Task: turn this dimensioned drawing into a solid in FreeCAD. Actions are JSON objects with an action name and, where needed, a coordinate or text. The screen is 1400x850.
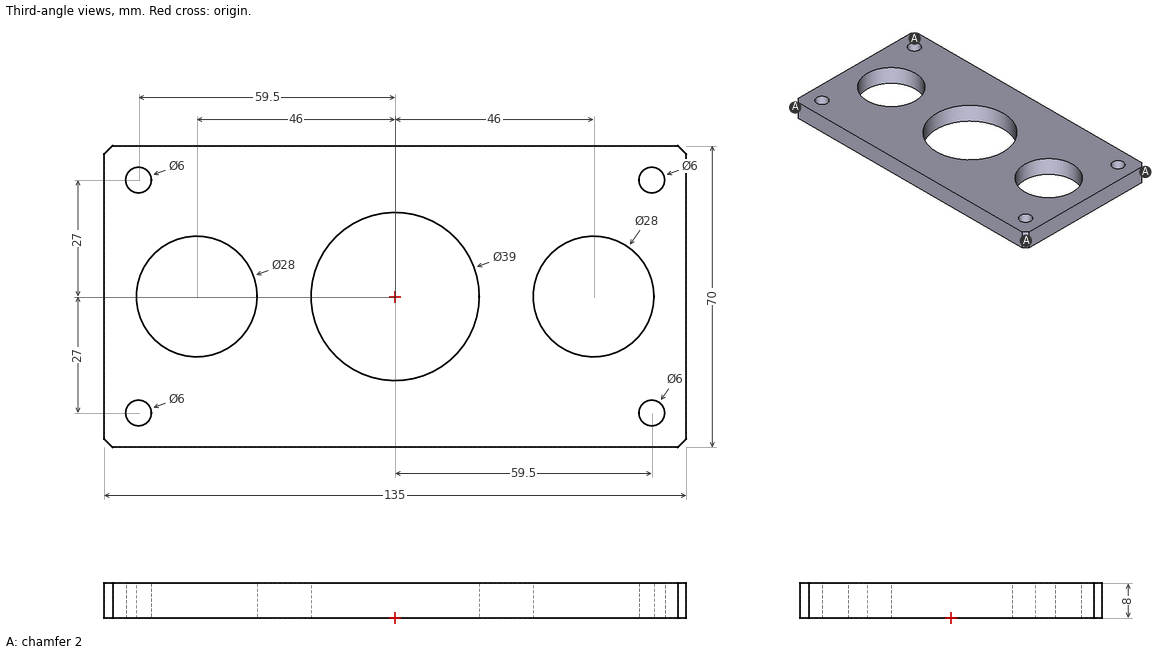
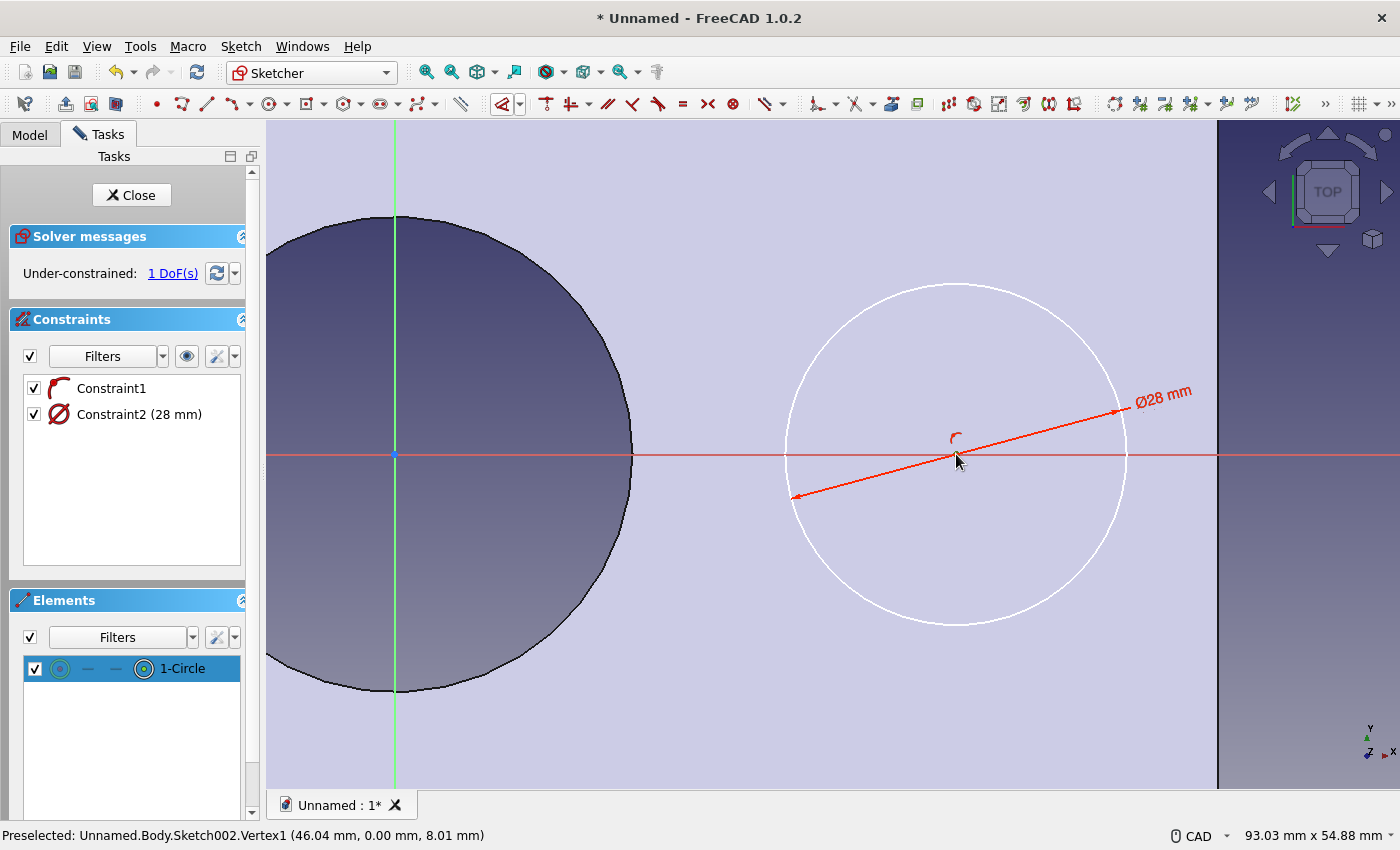
{"action": "key", "text": "l"}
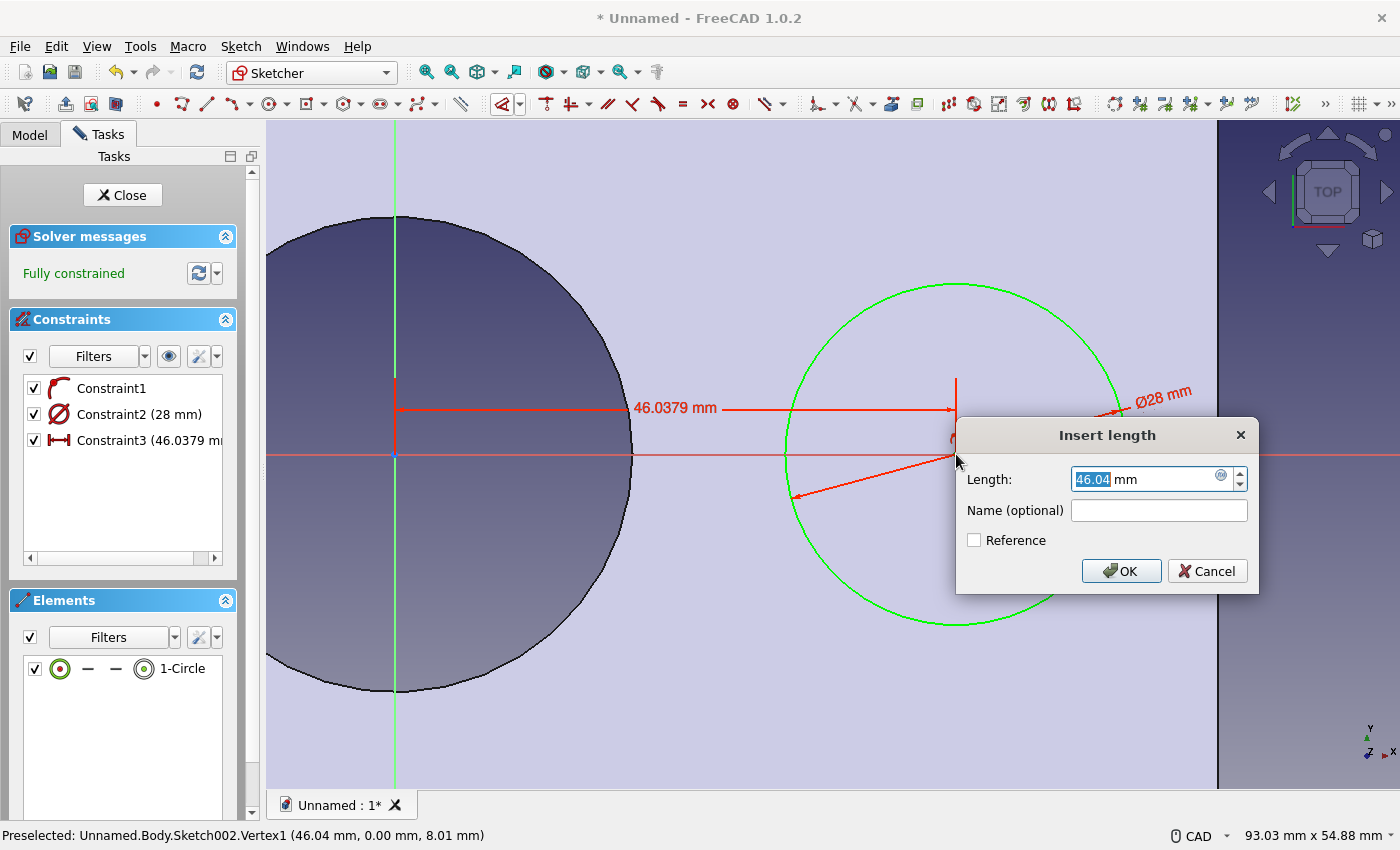
{"action": "type", "text": "46"}
{"action": "key", "text": "Return"}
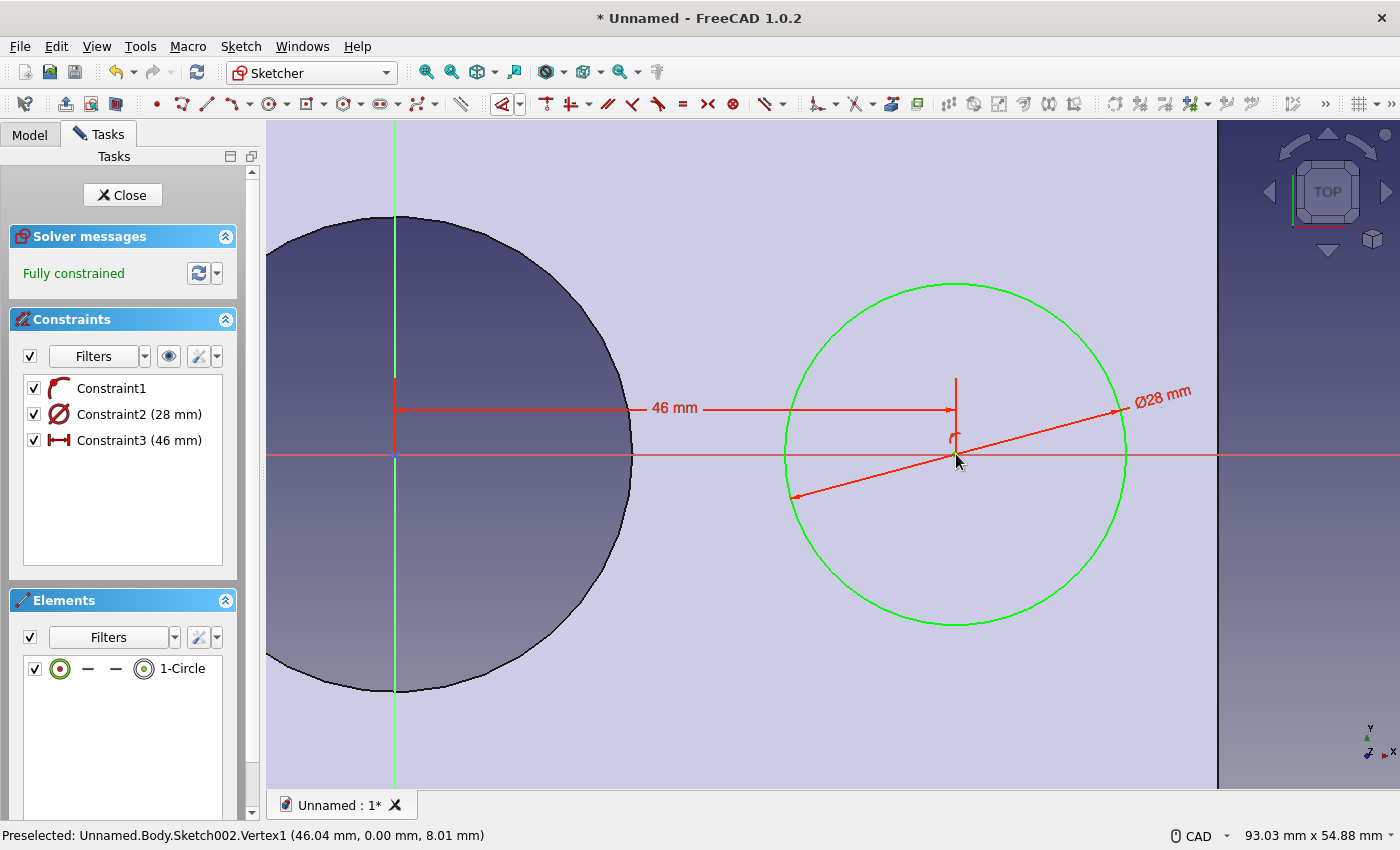
{"action": "left_click", "coordinate": [123, 195]}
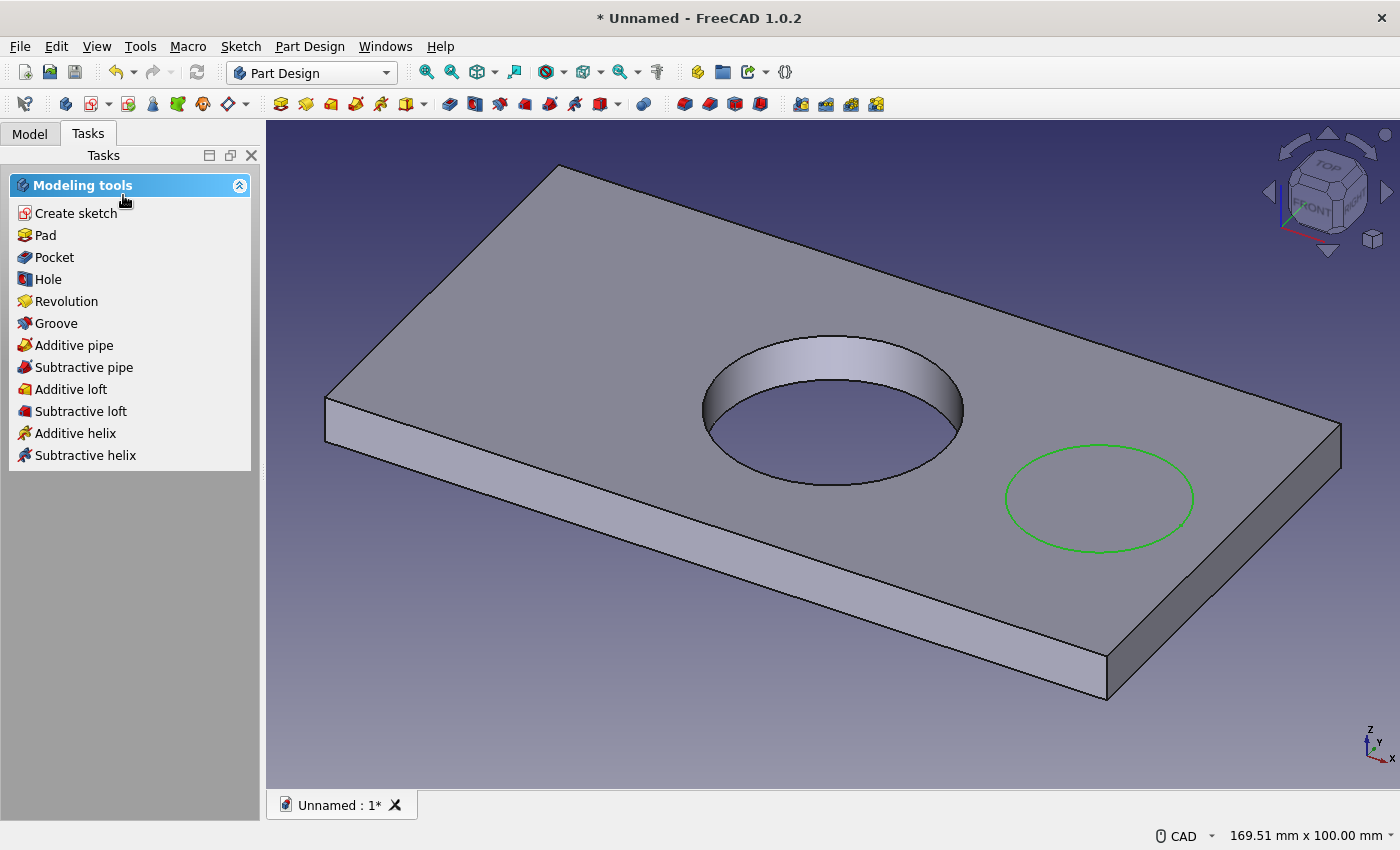
{"action": "left_click", "coordinate": [450, 104]}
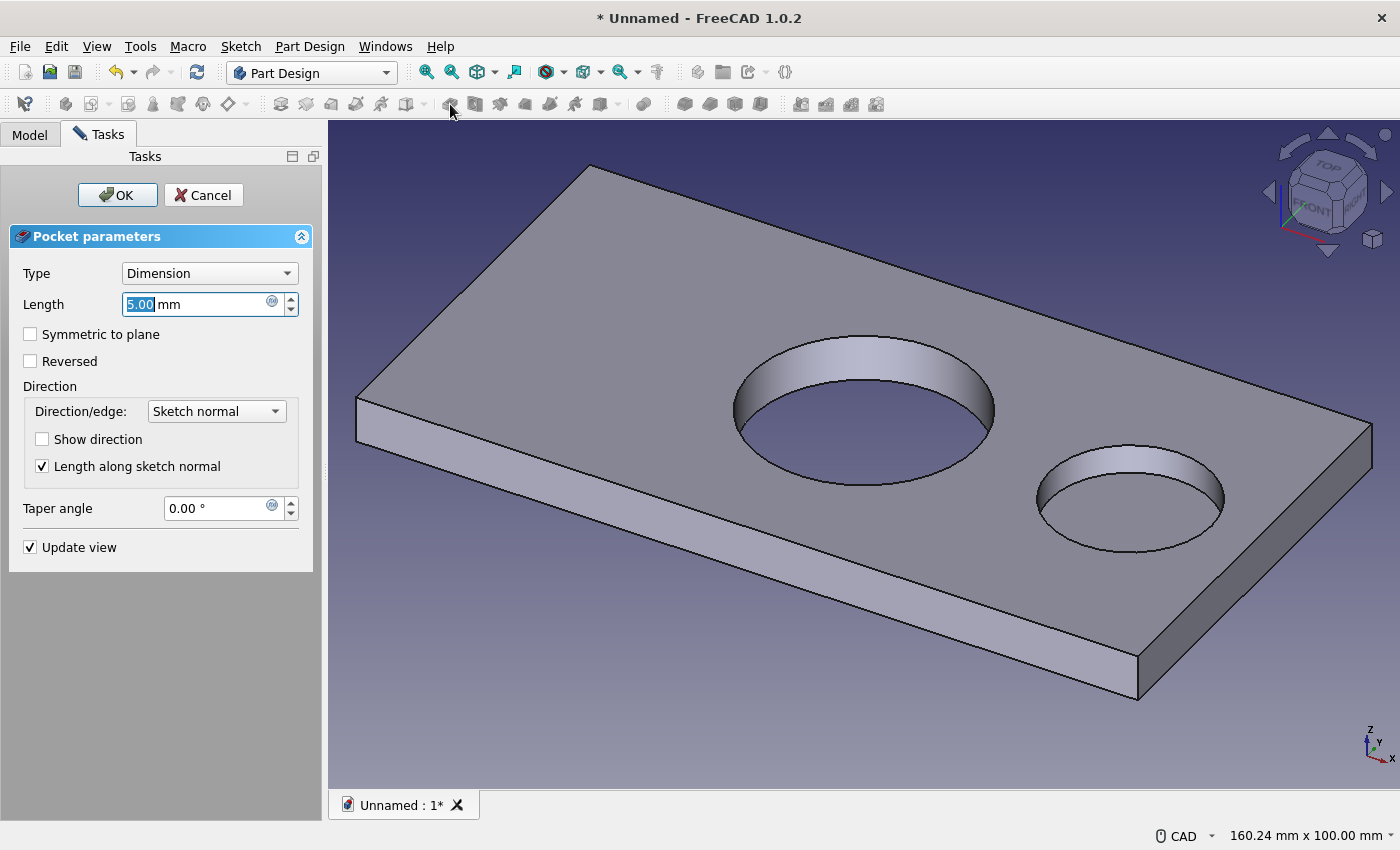
{"action": "left_click", "coordinate": [210, 274]}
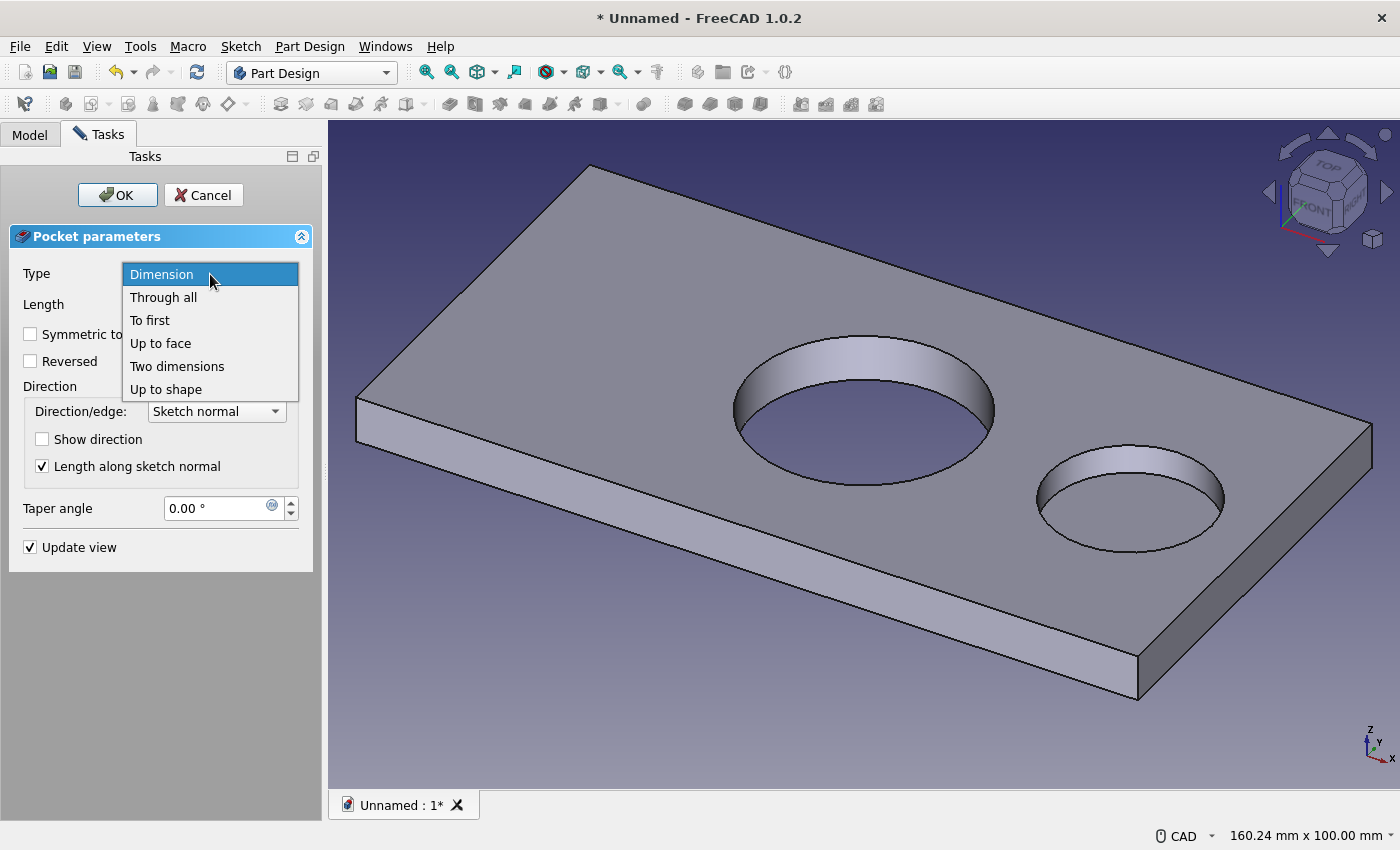
{"action": "left_click", "coordinate": [208, 320]}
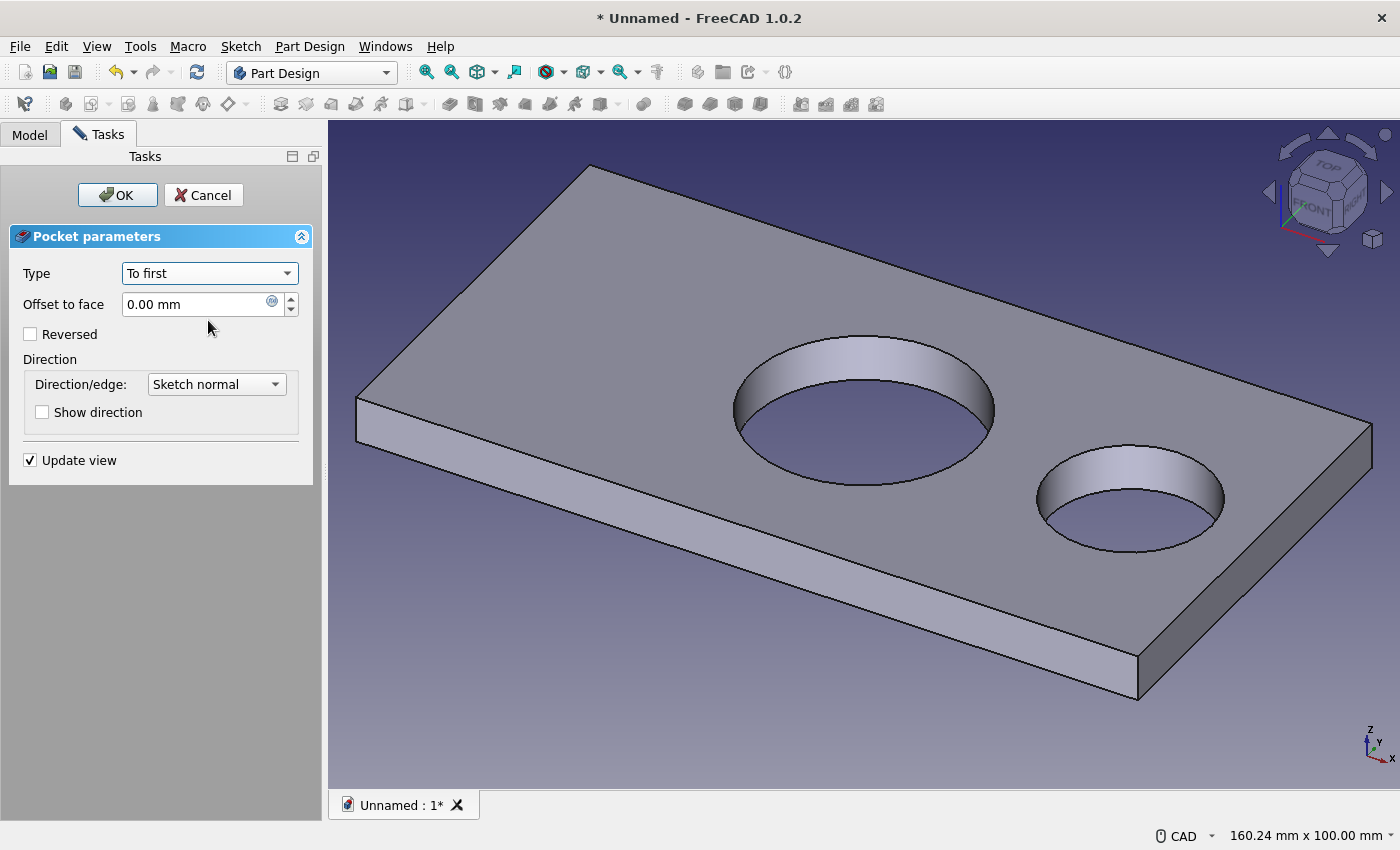
{"action": "left_click", "coordinate": [118, 195]}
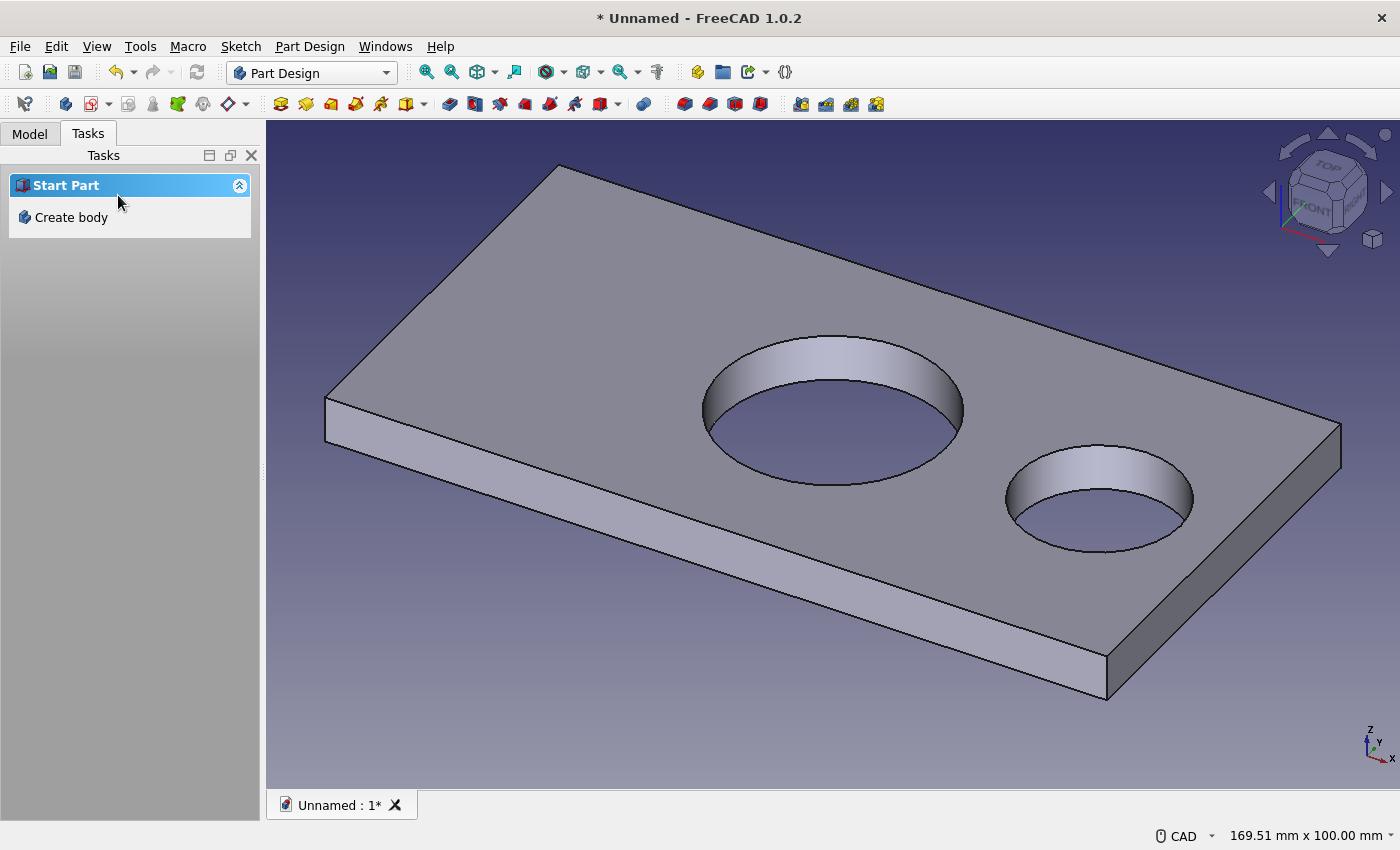
{"action": "left_click", "coordinate": [576, 369]}